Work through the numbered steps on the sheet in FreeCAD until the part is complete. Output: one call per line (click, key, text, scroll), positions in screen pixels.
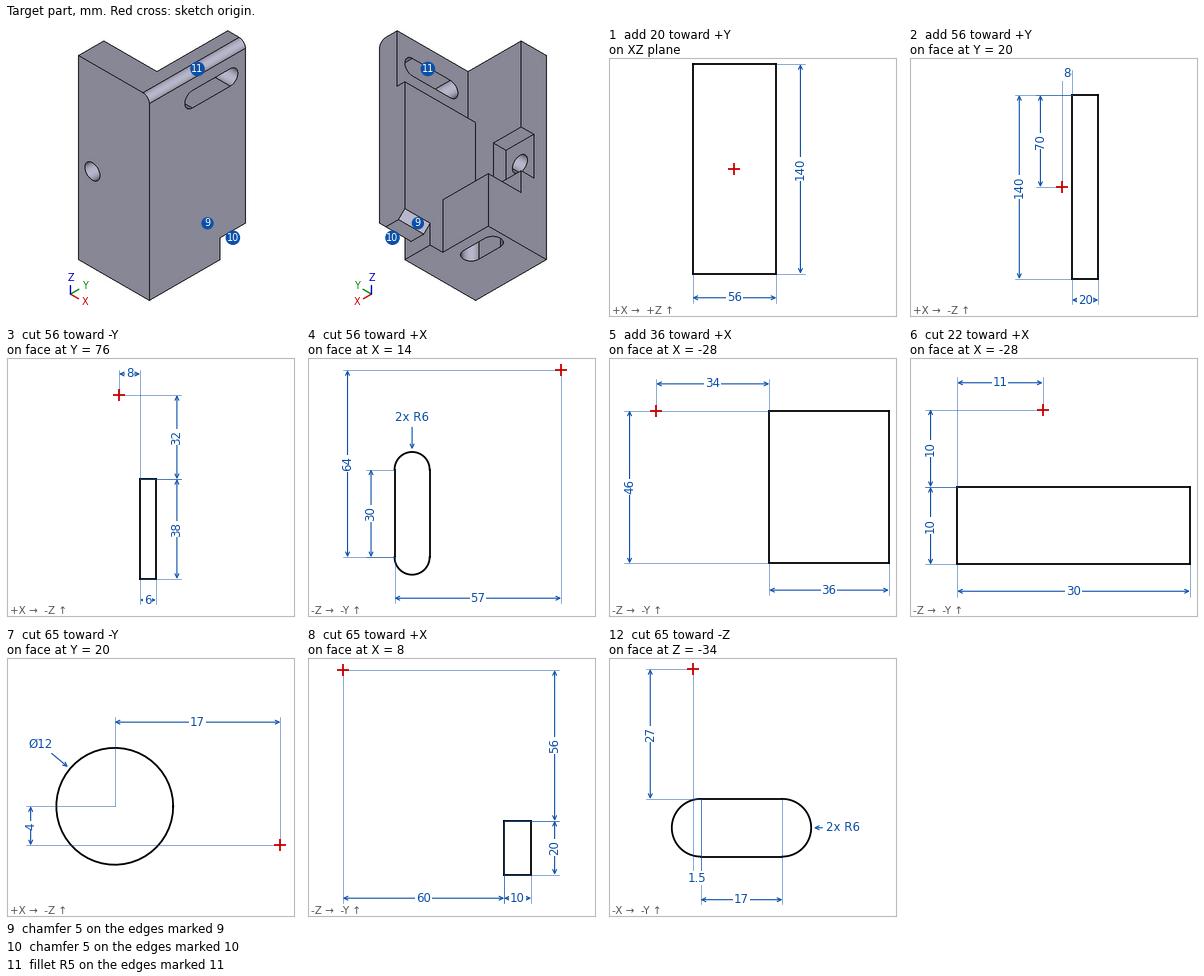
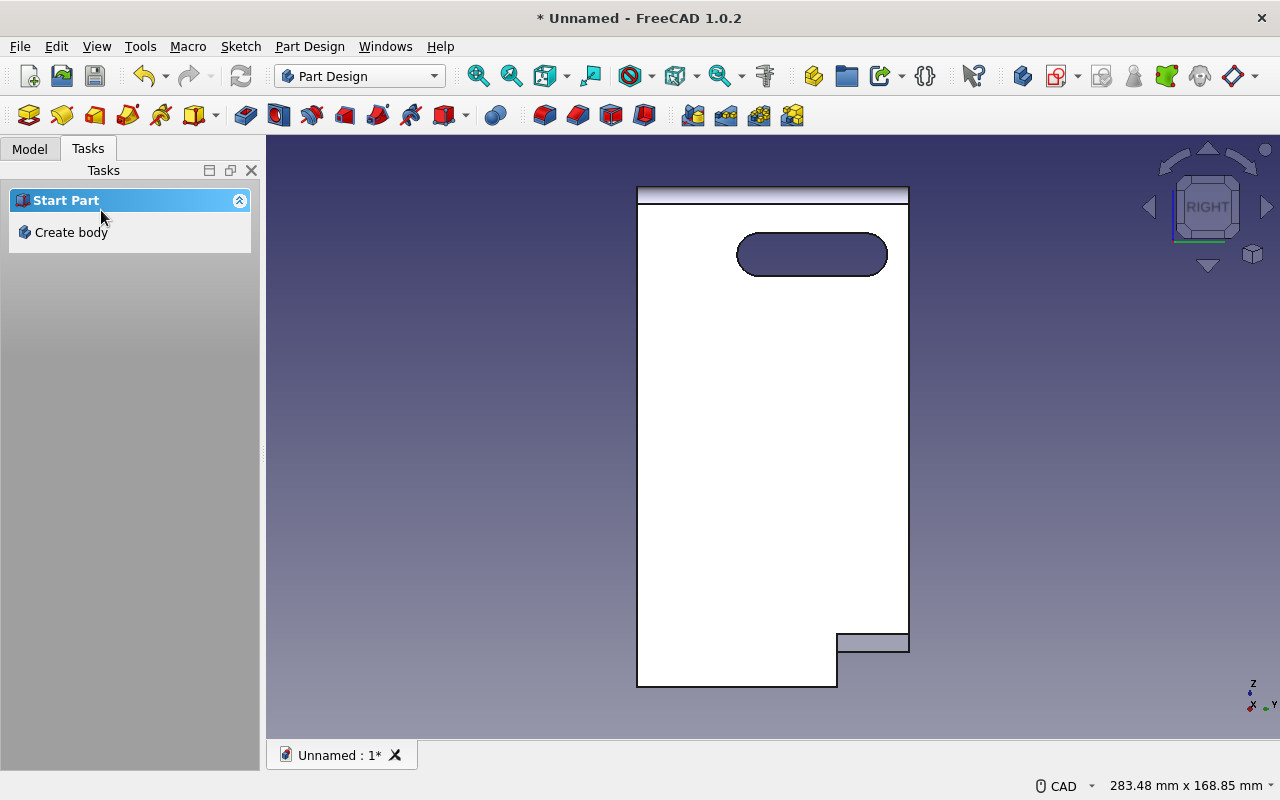
key(0)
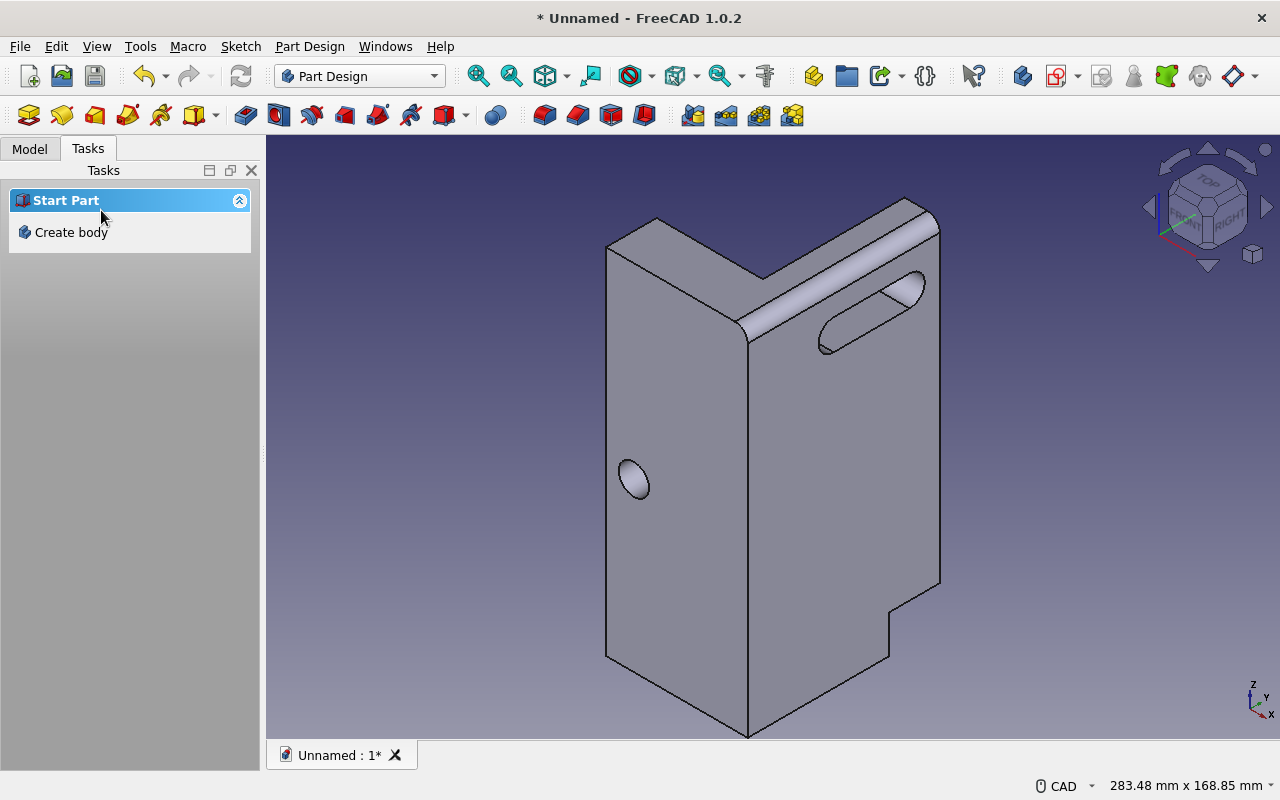
key(2)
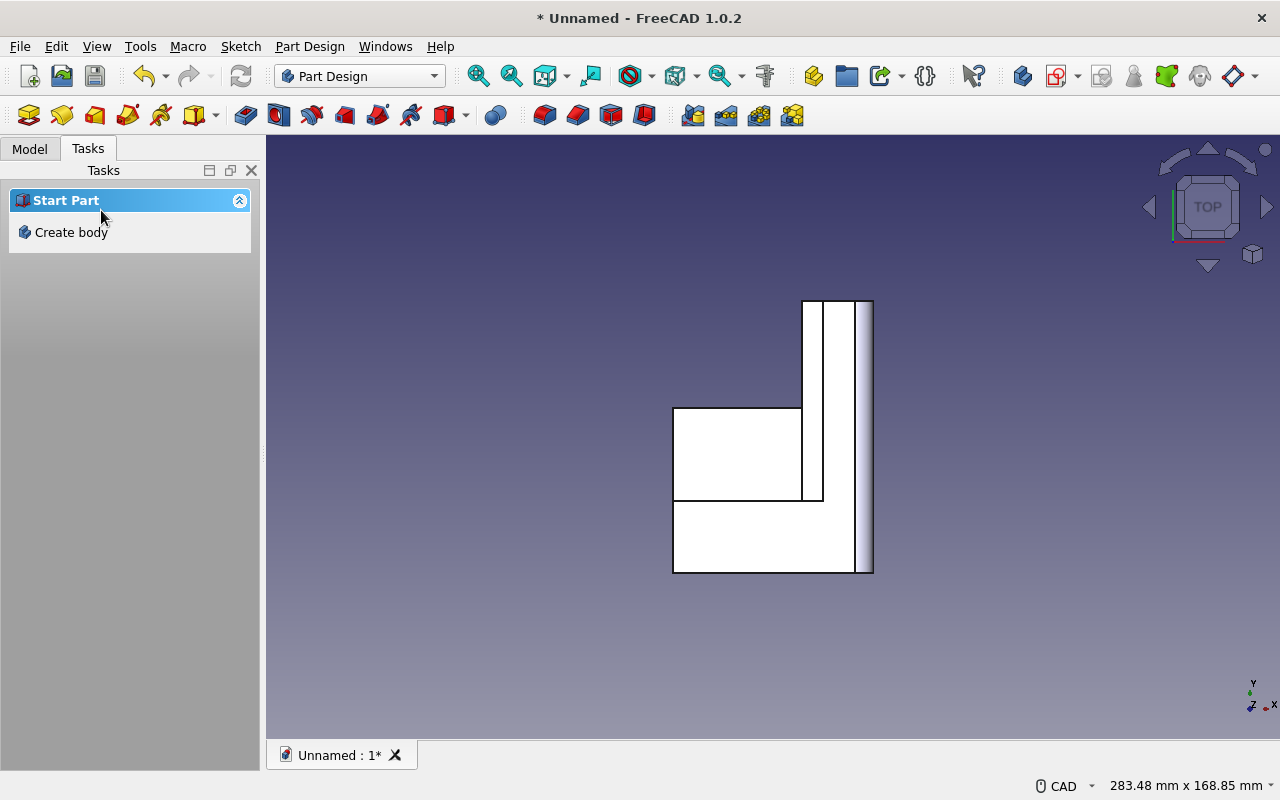
click(737, 454)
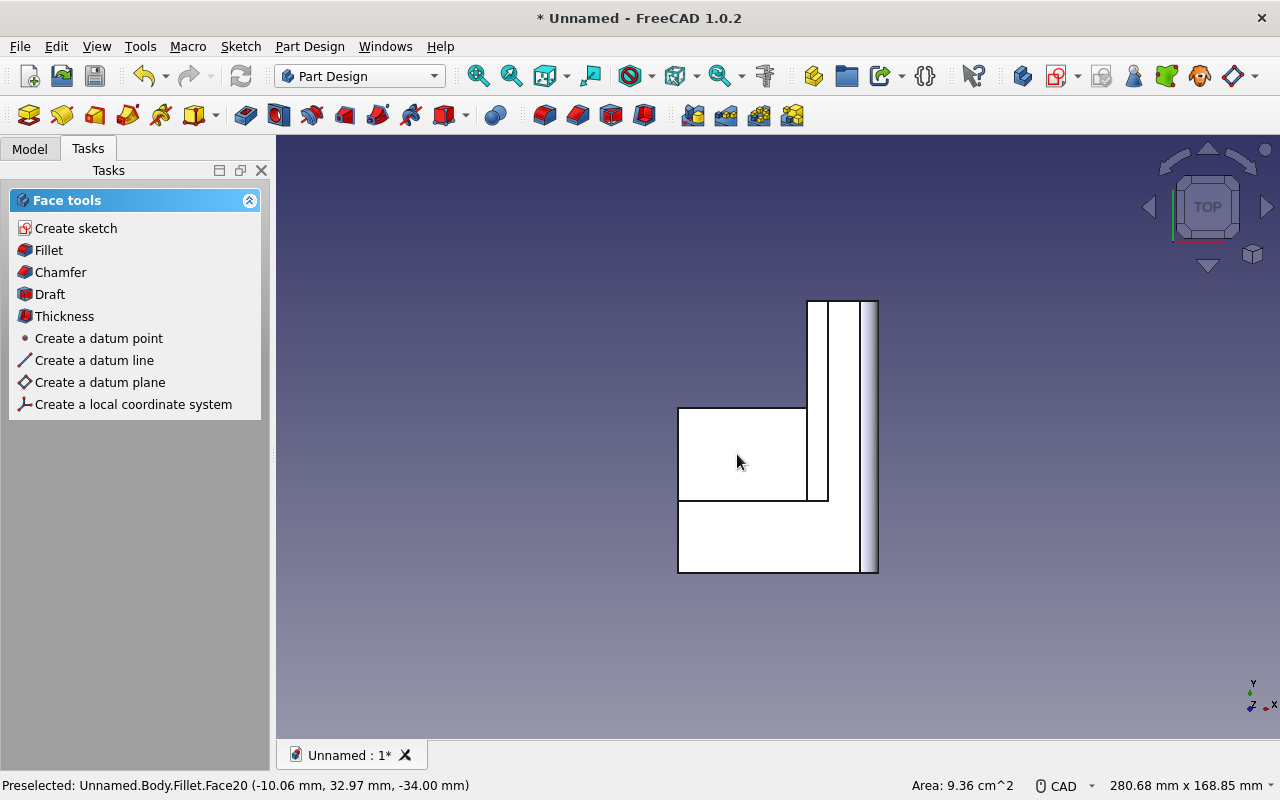
click(1056, 76)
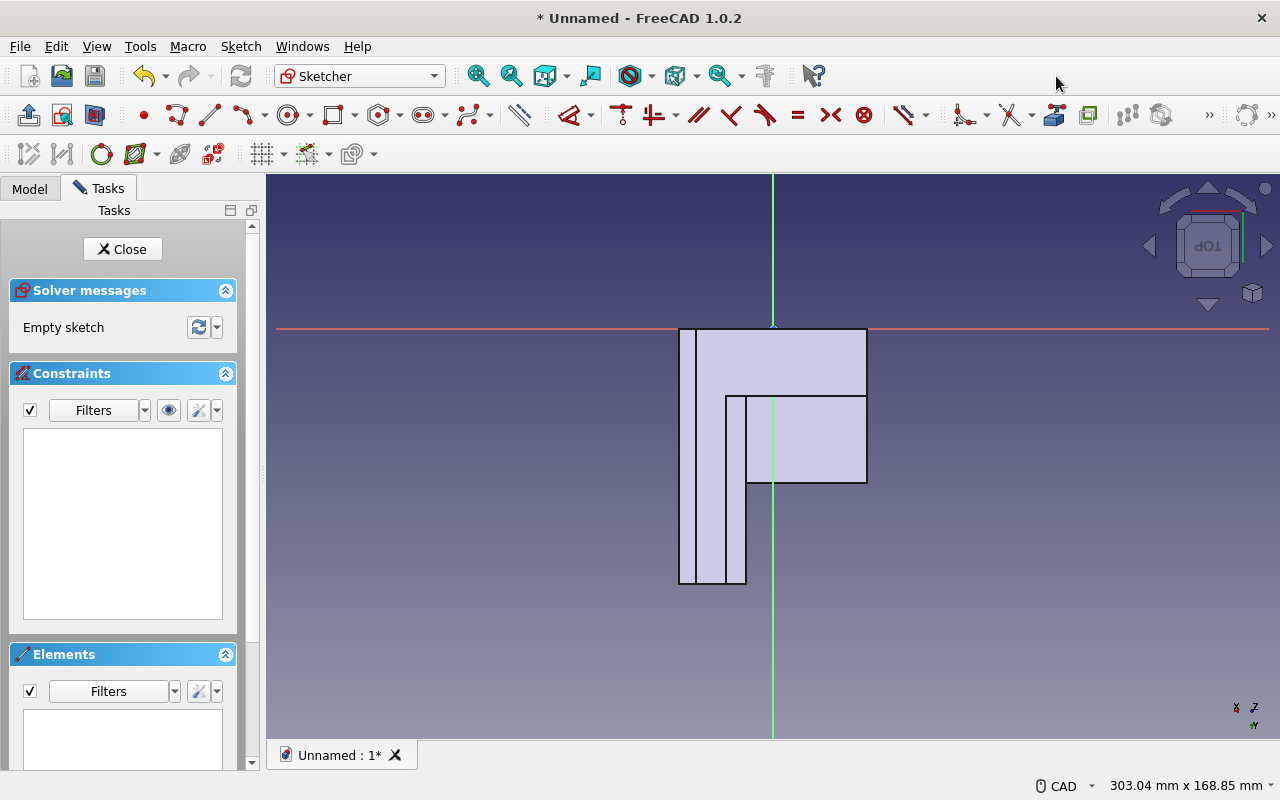
scroll(866, 359, up, 5)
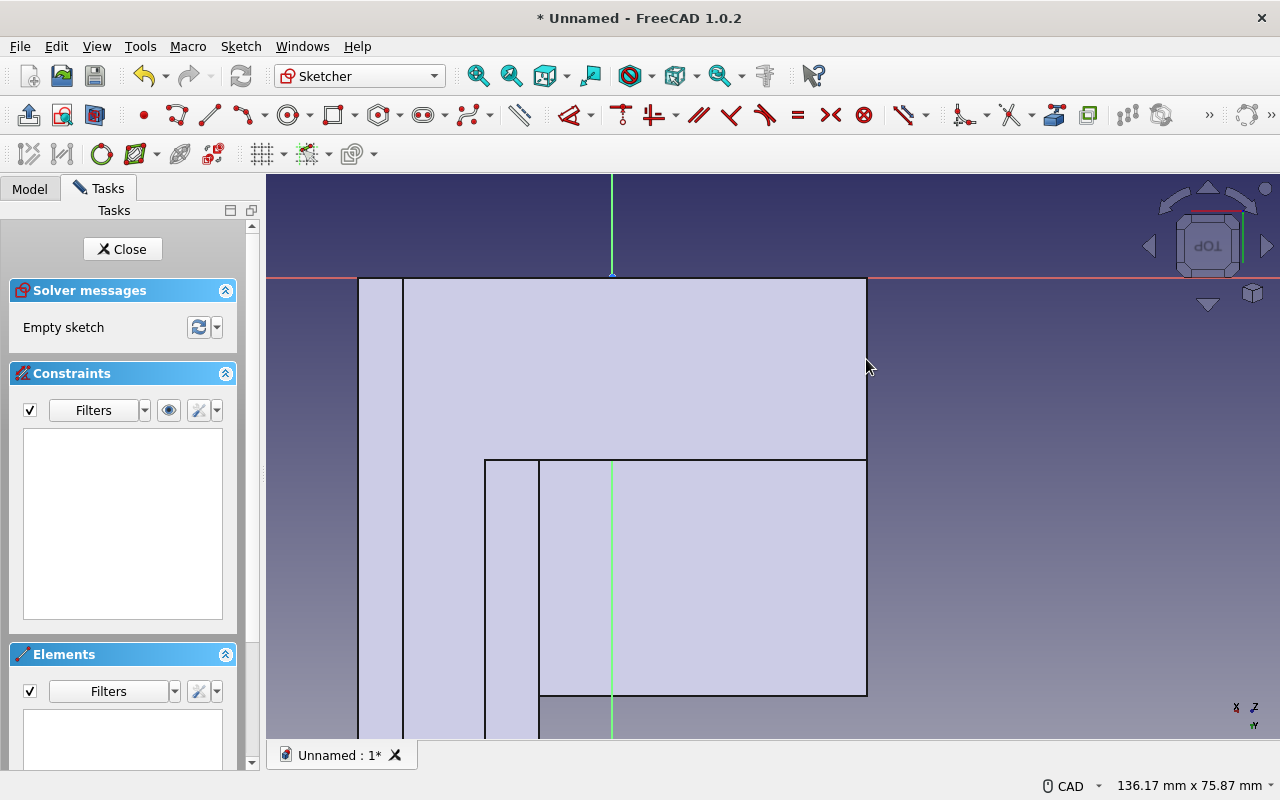
key(g)
key(s)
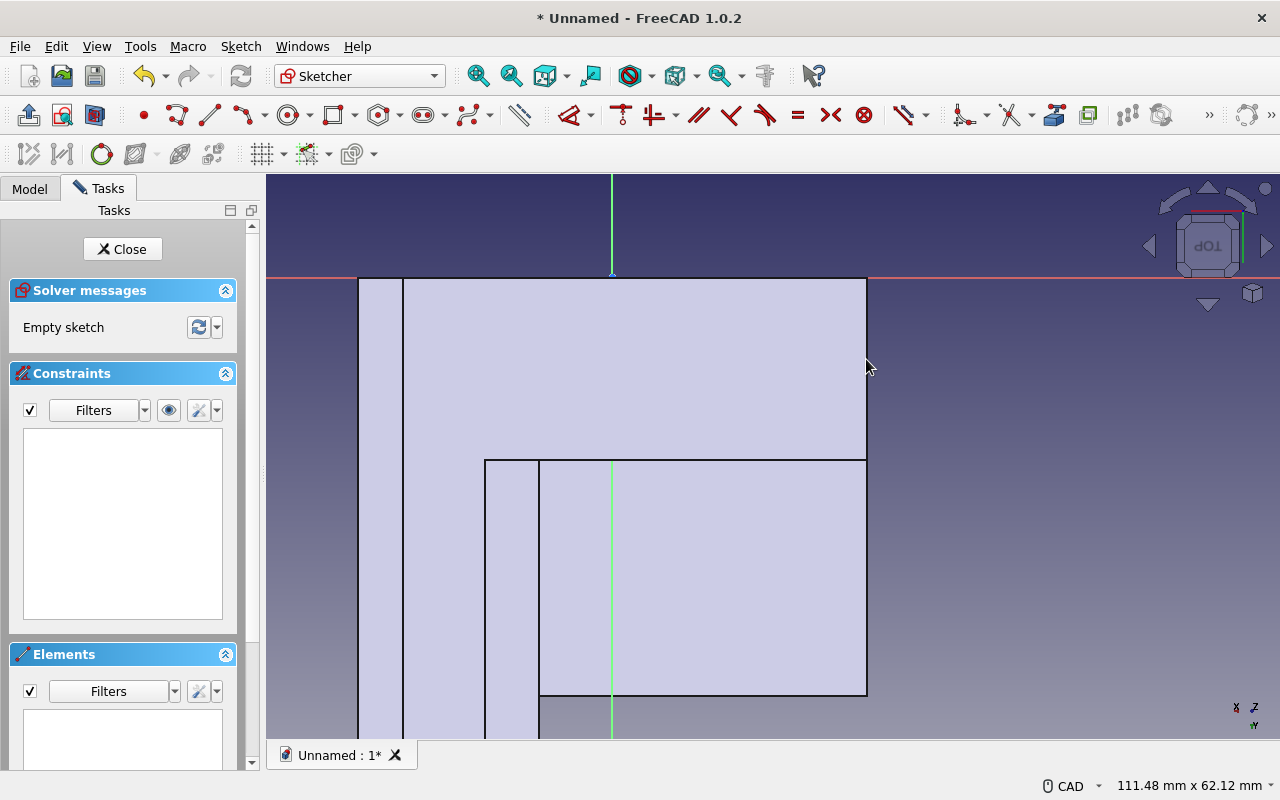
click(626, 578)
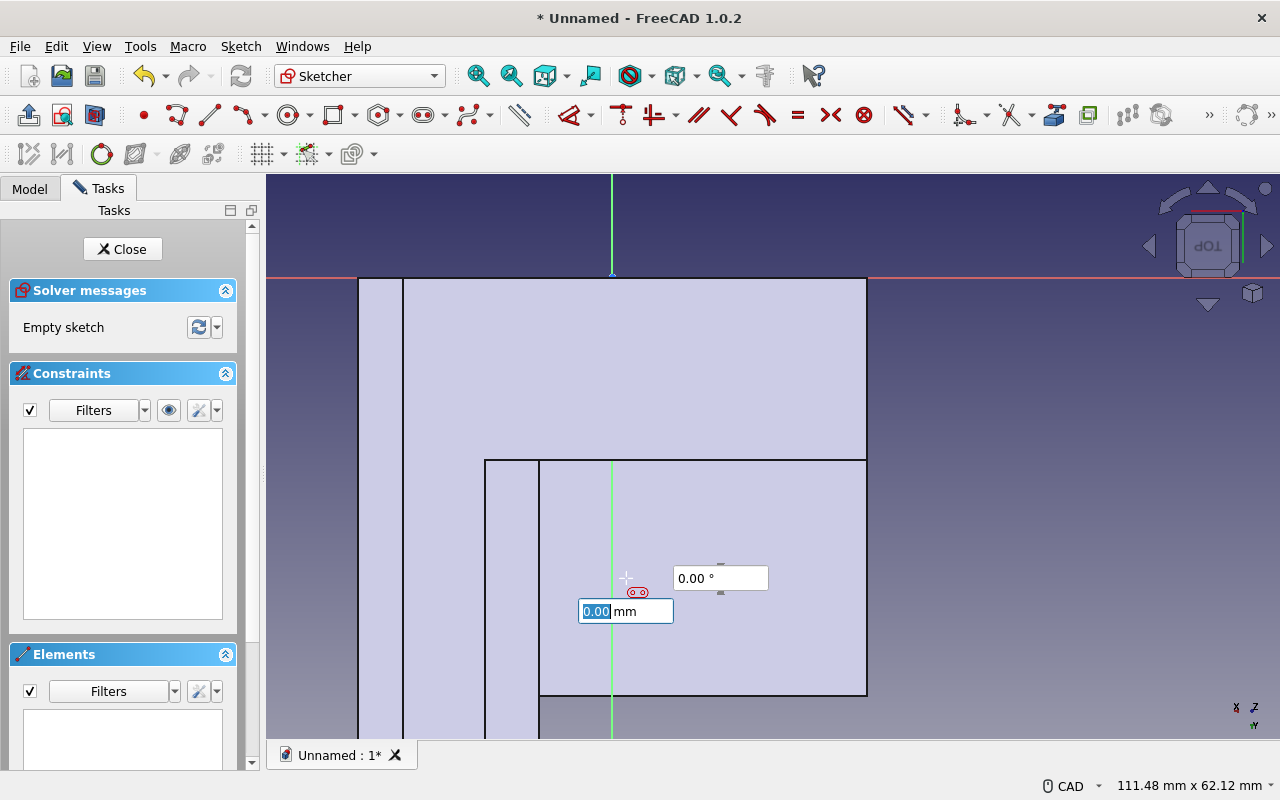
click(780, 578)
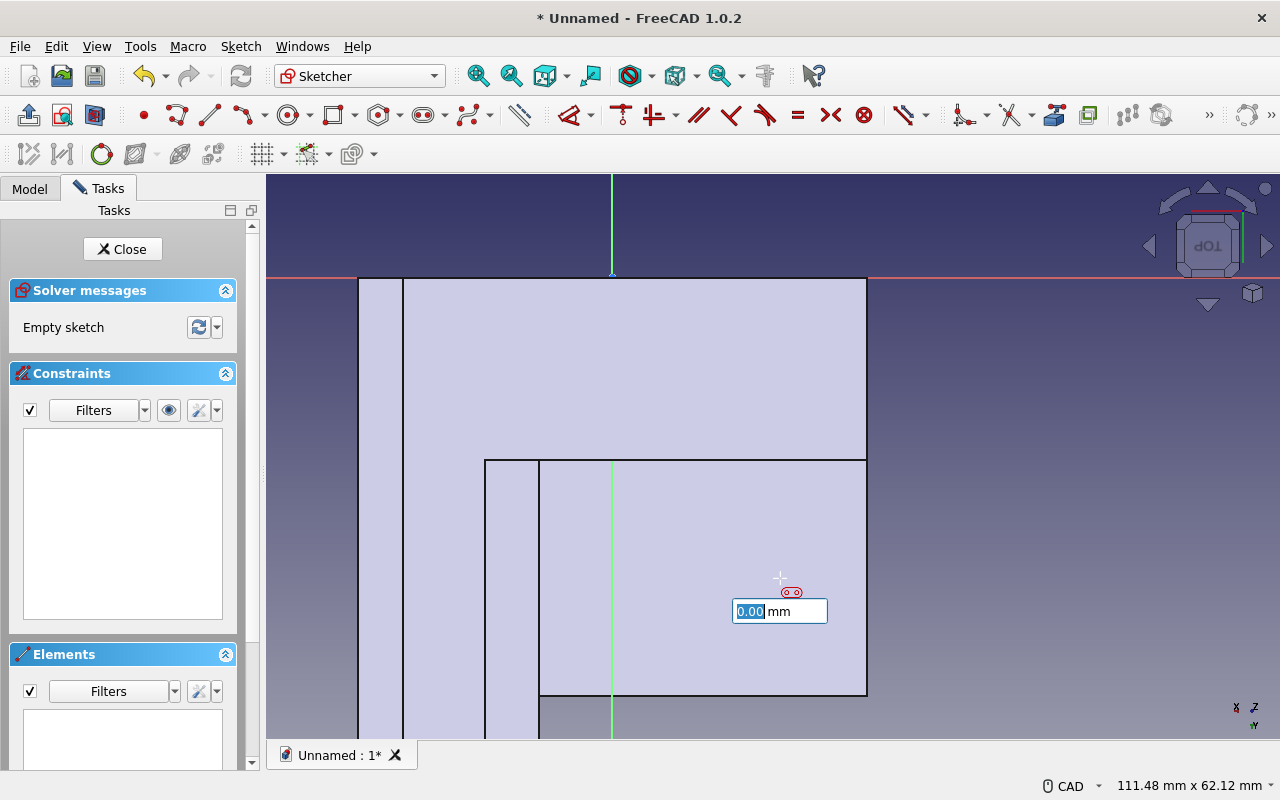
click(703, 633)
key(Escape)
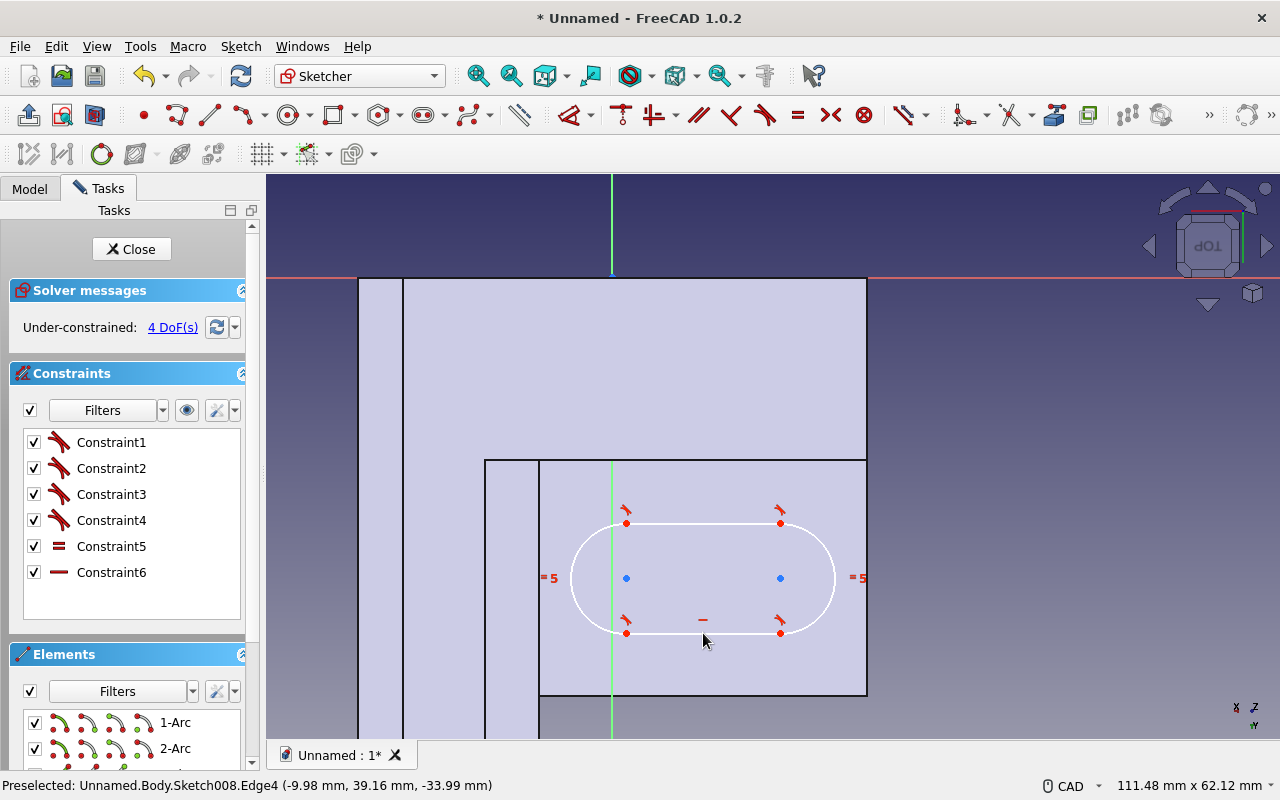
click(568, 116)